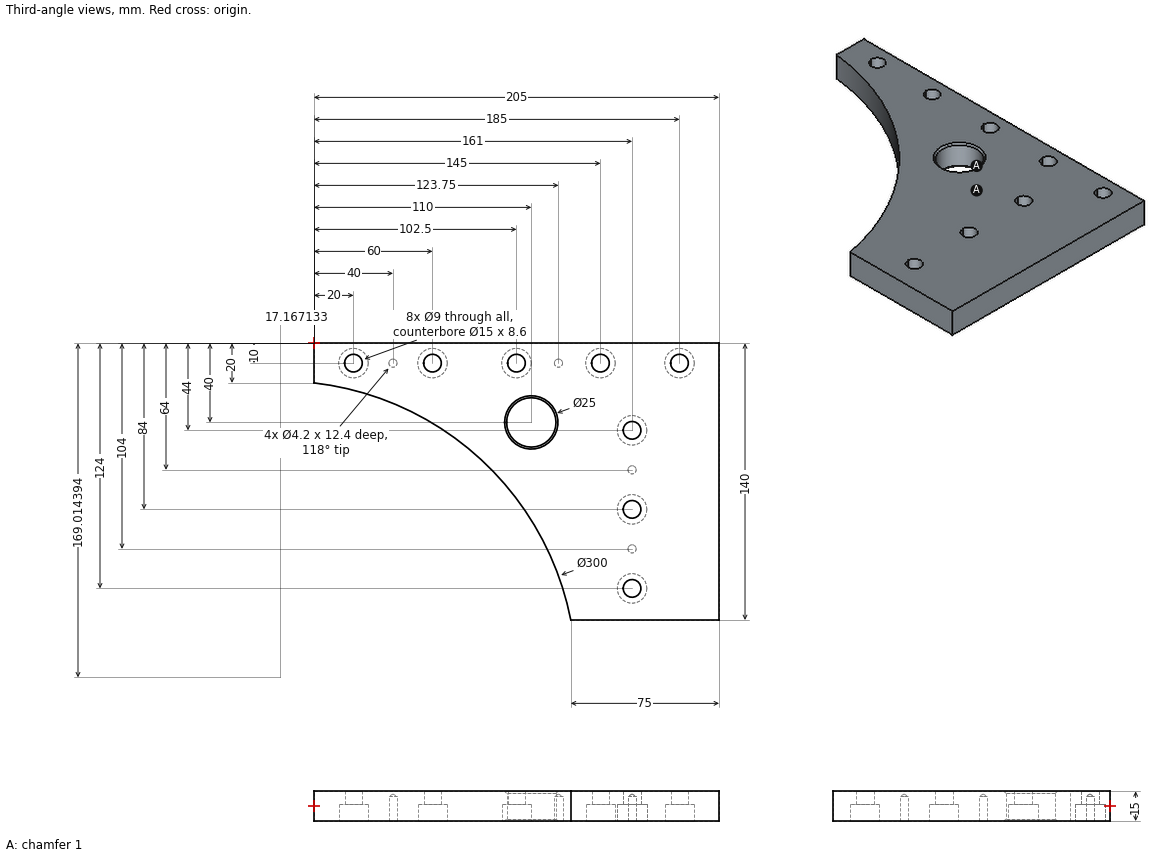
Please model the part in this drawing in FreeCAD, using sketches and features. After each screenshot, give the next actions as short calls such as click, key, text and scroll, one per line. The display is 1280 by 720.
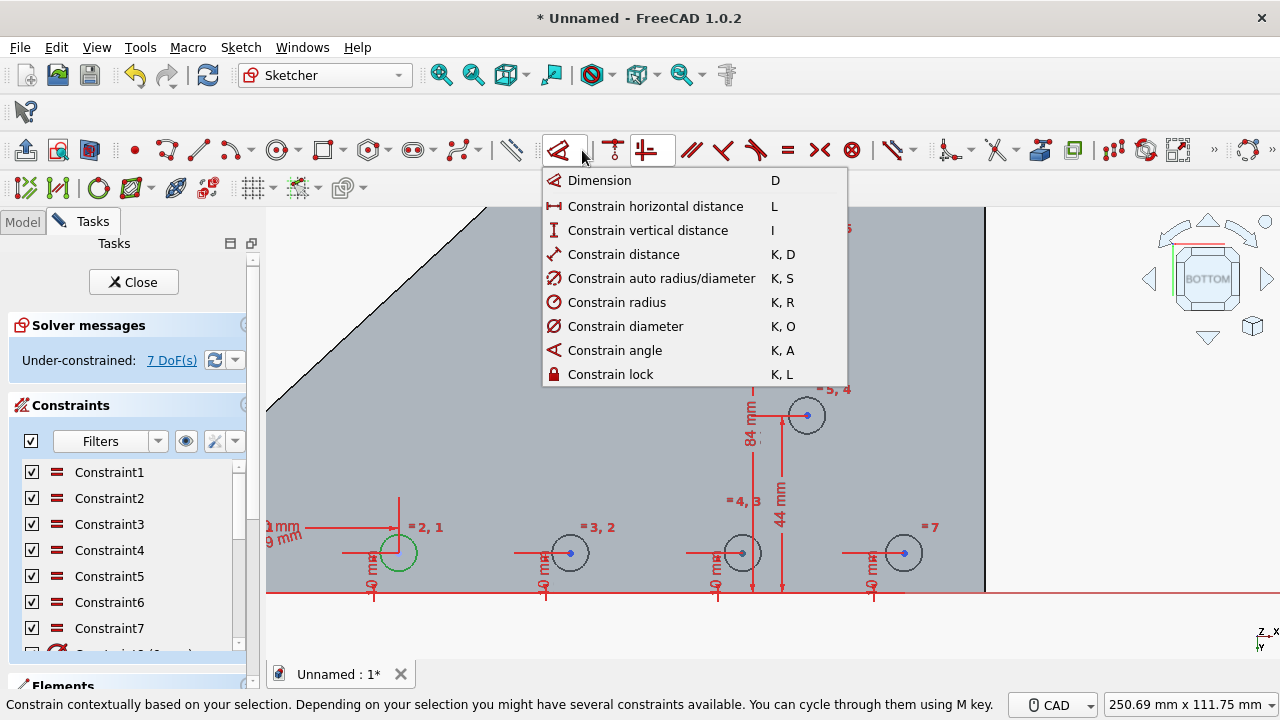
click(695, 206)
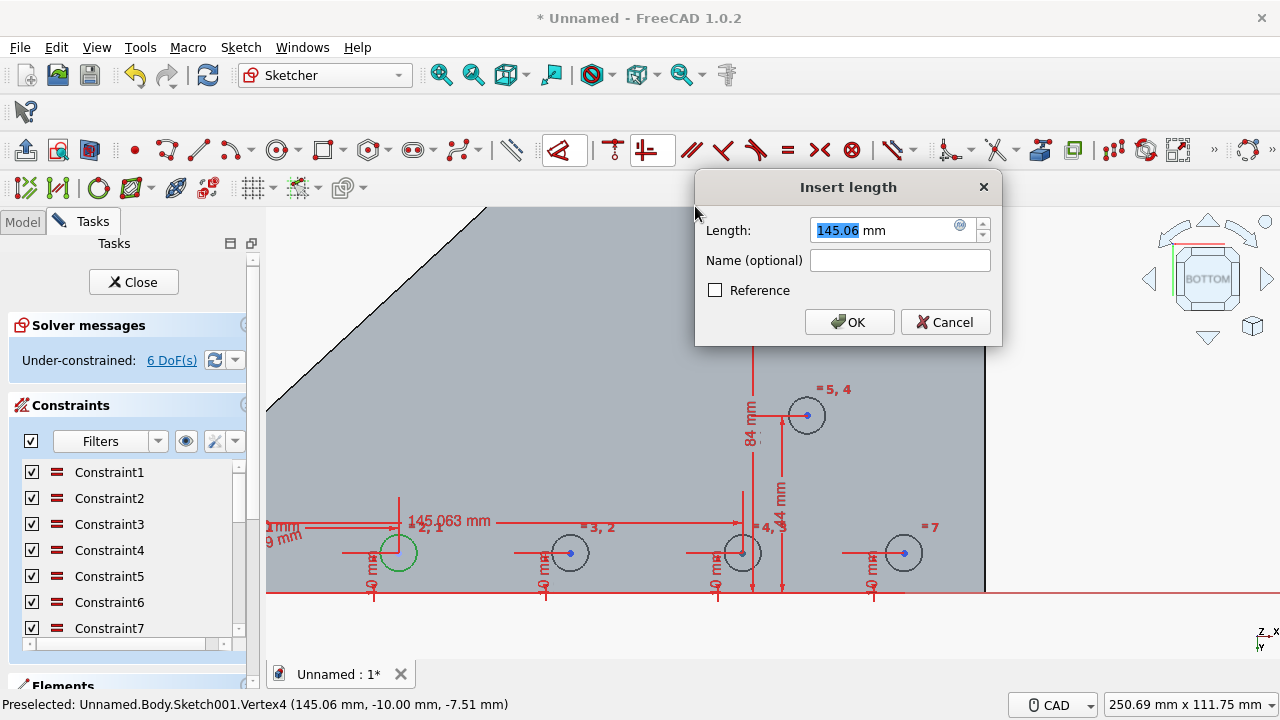
text(145)
key(Return)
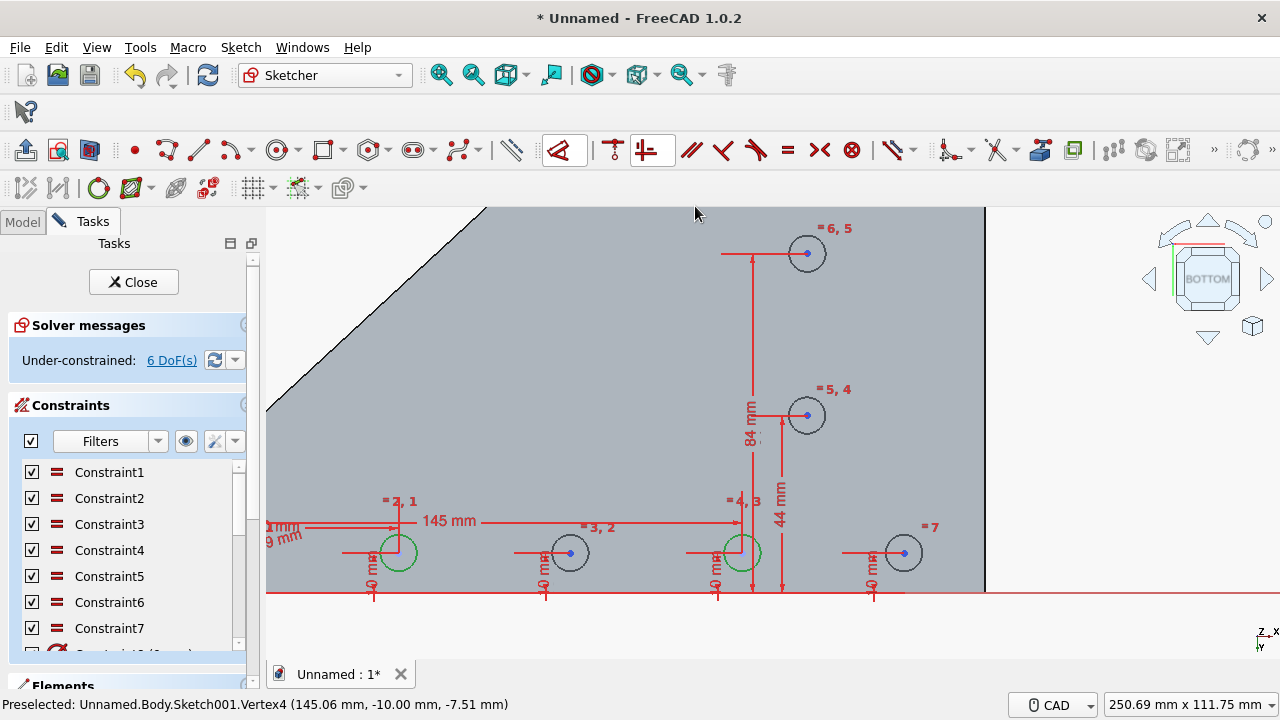
click(807, 416)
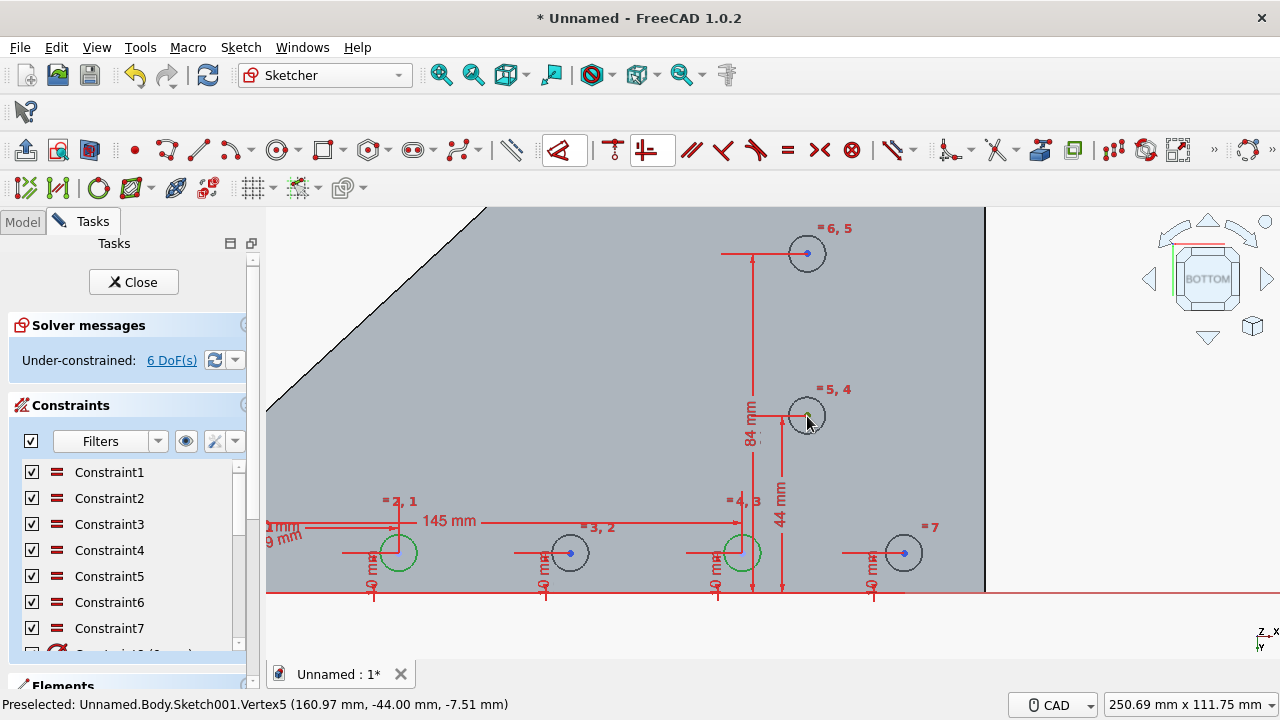
click(582, 150)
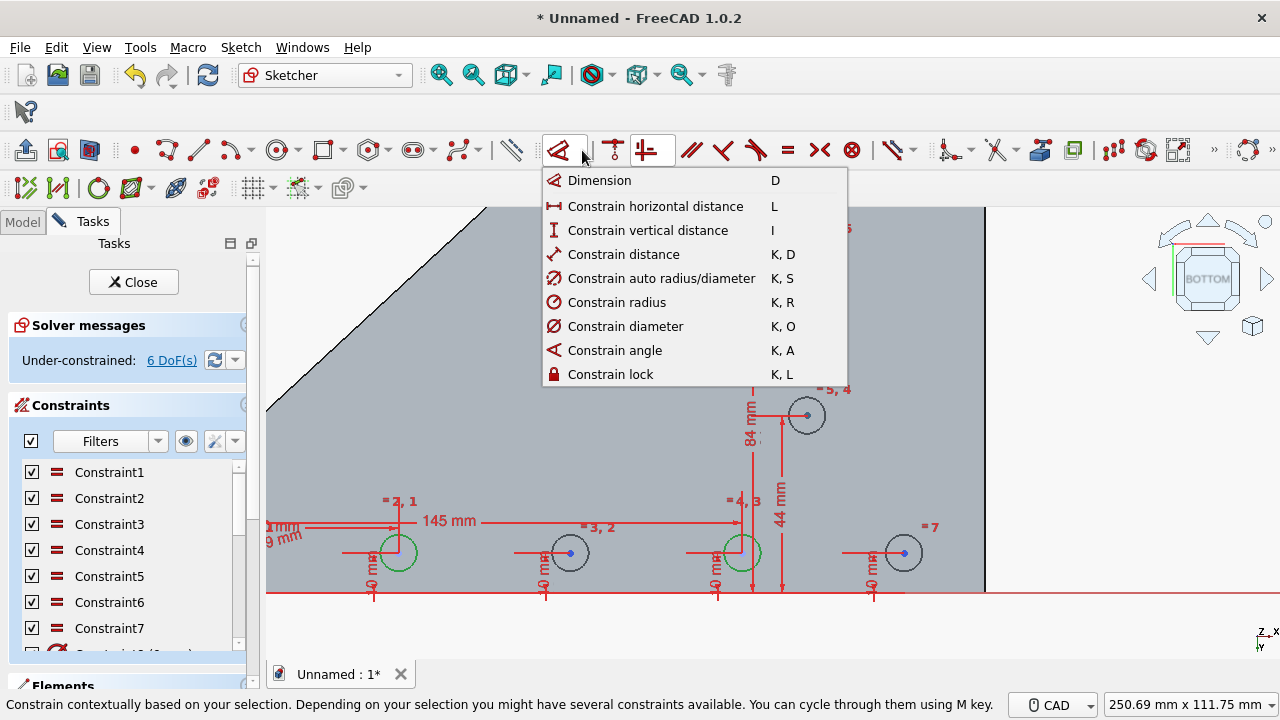
click(695, 206)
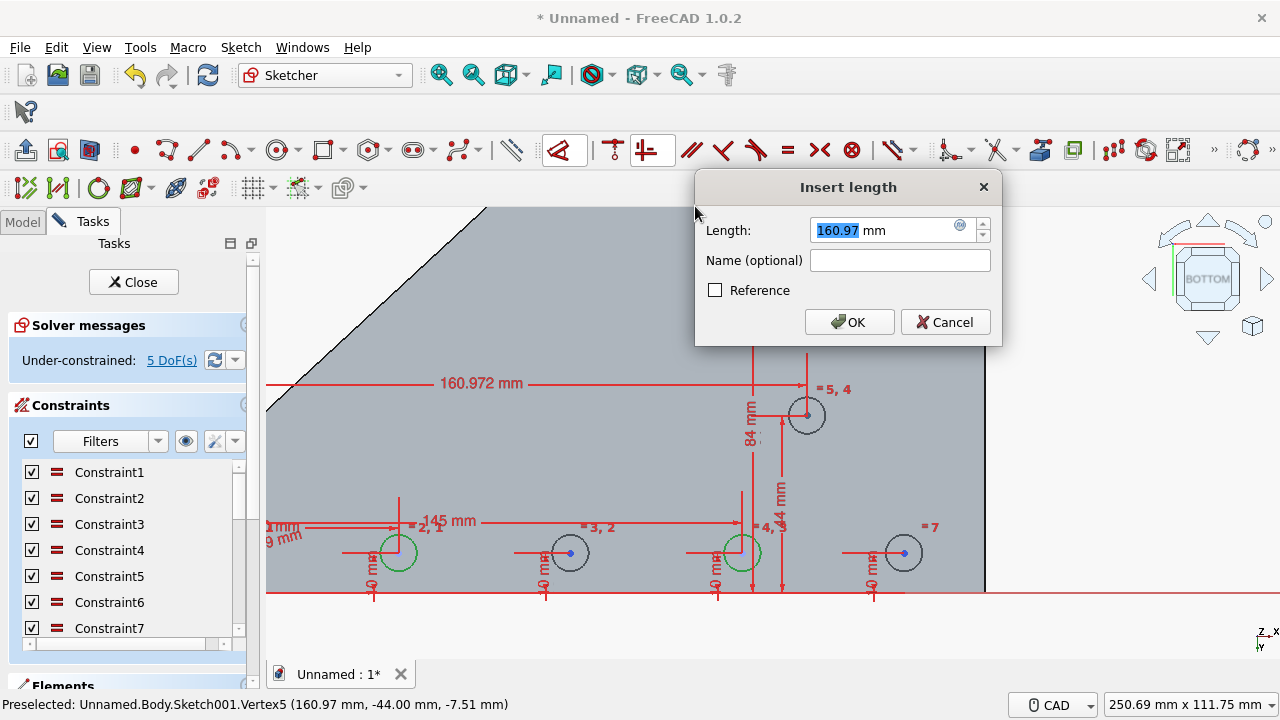
text(161)
key(Return)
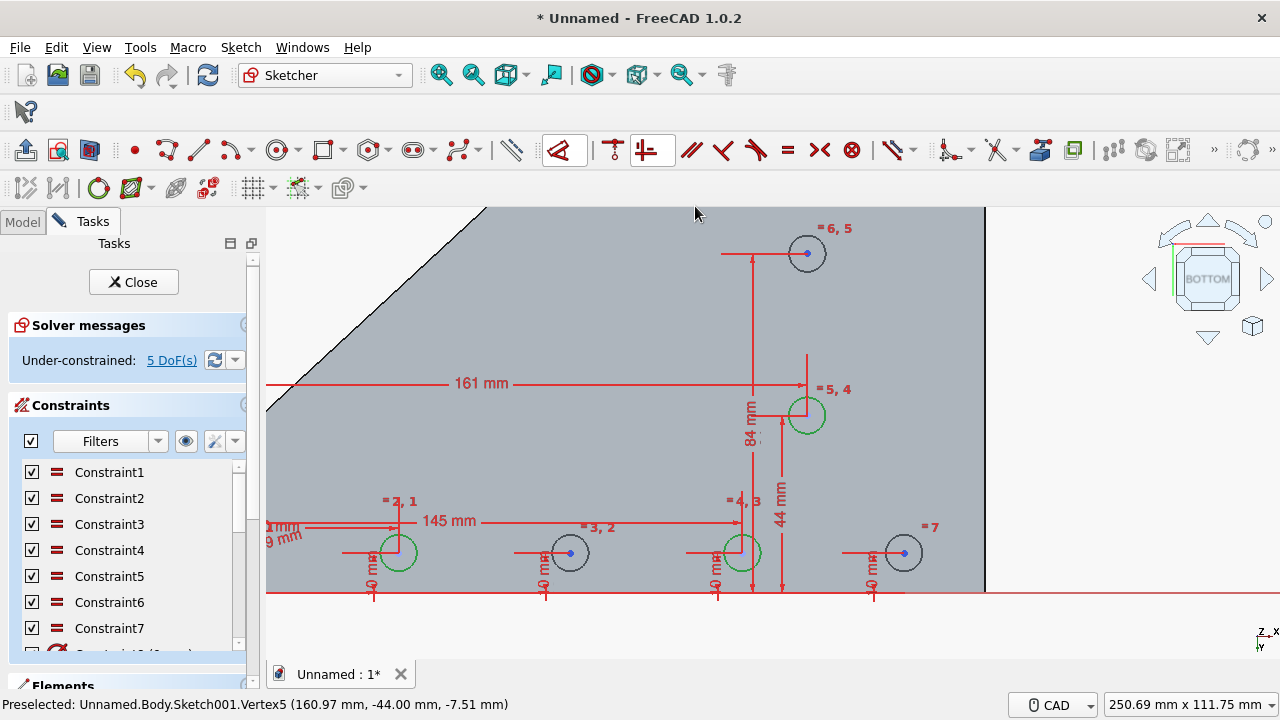
click(807, 254)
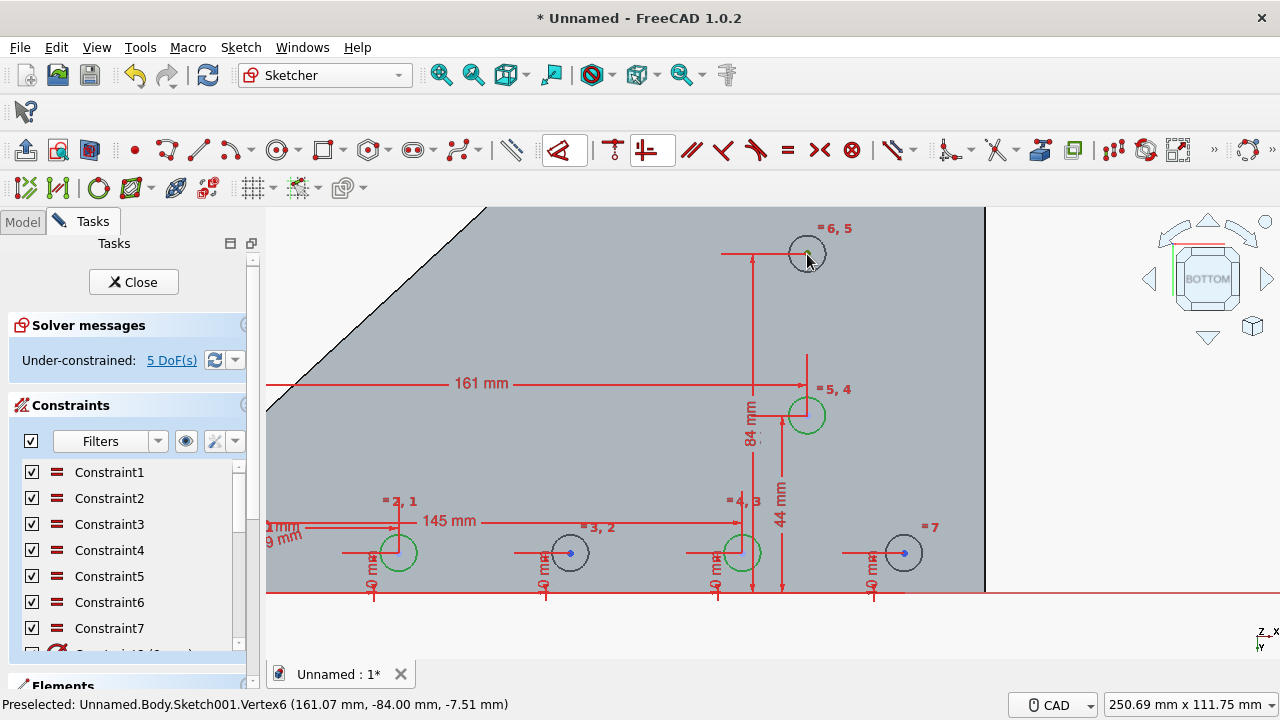
click(582, 150)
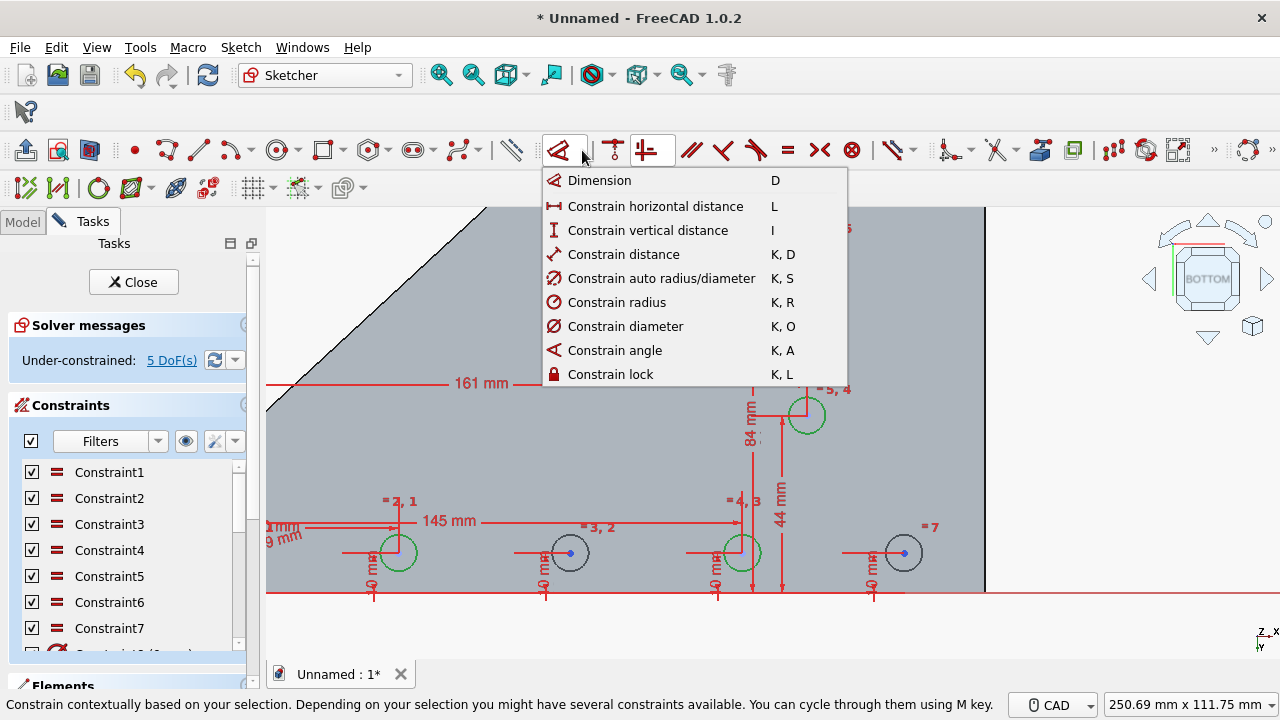
click(695, 206)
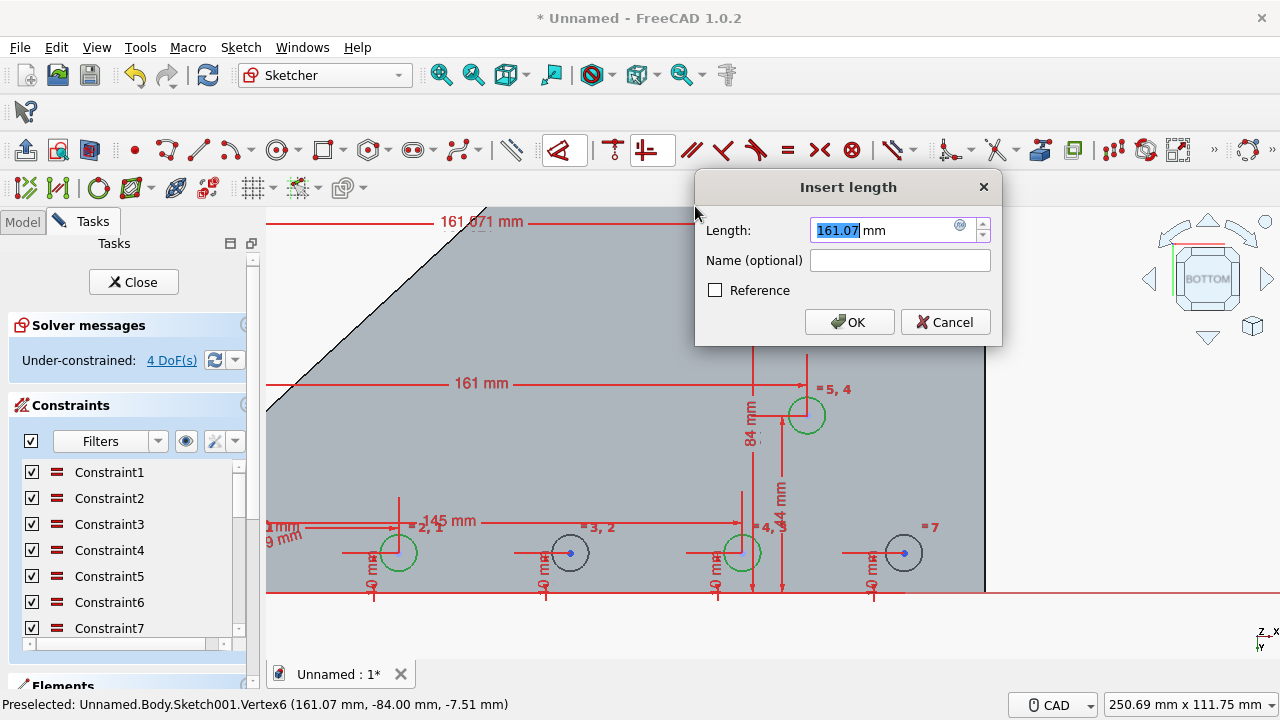
text(161)
key(Return)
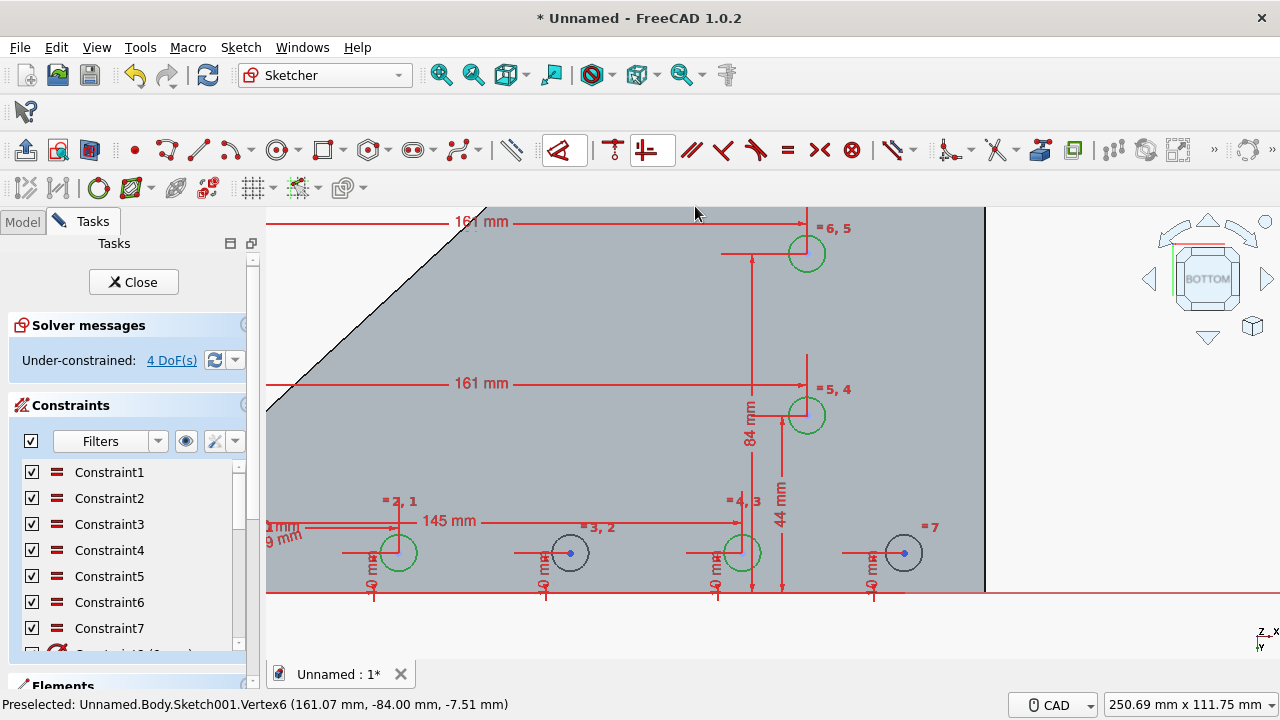
scroll(906, 554, down, 3)